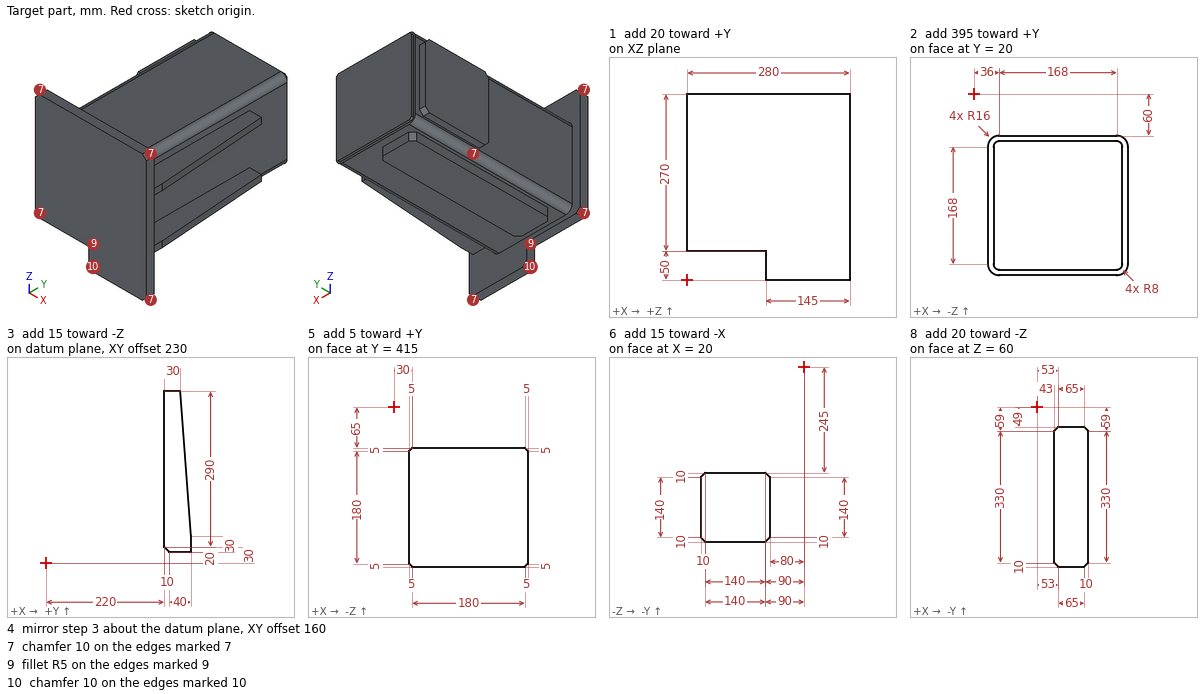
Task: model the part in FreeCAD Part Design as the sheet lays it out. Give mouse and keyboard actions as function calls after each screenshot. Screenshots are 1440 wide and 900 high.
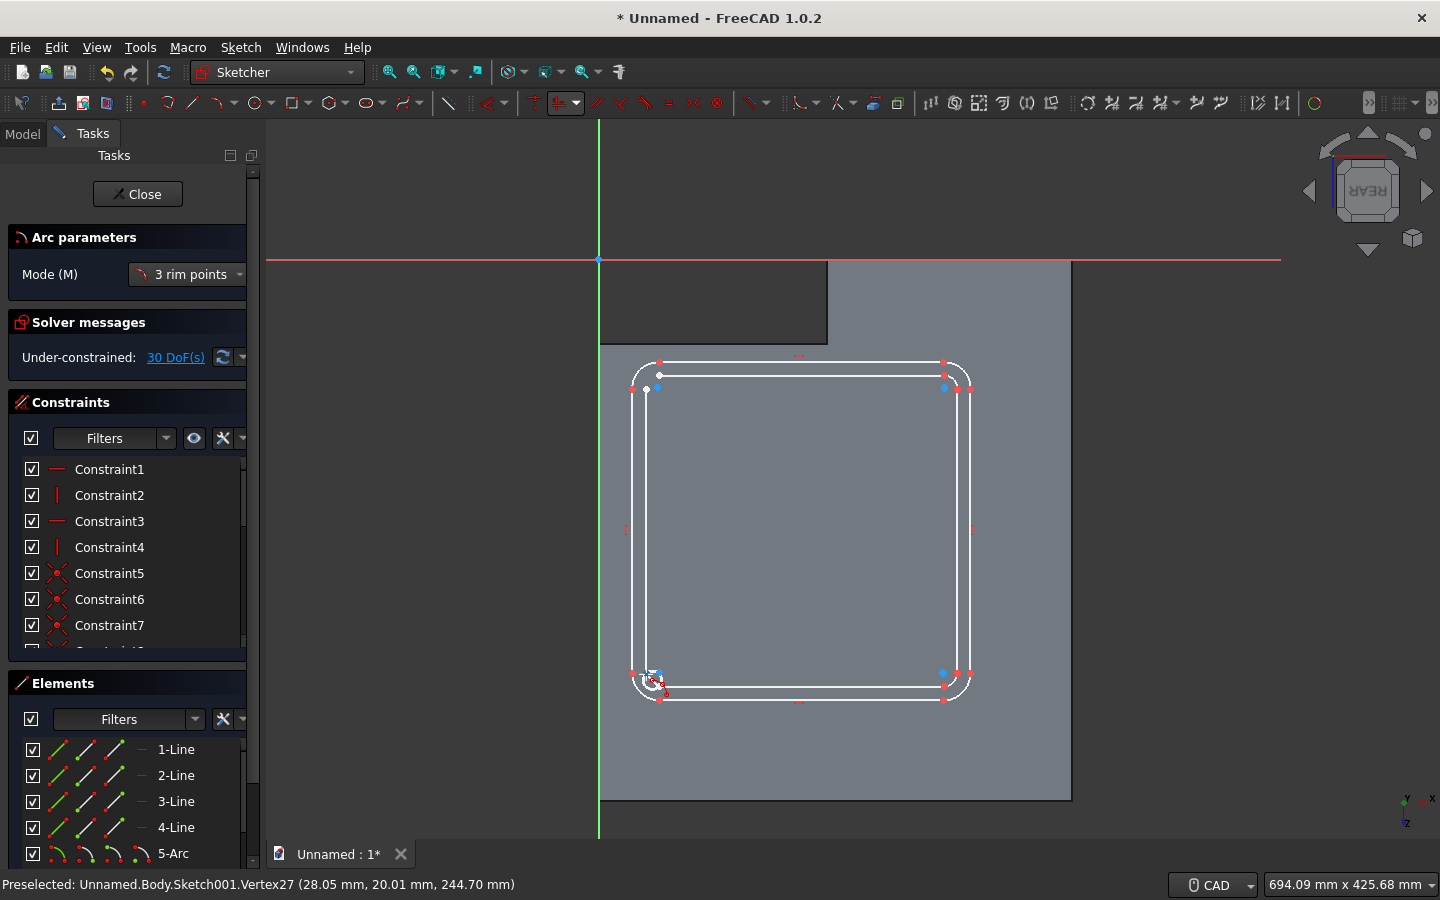
scroll(650, 682, up, 7)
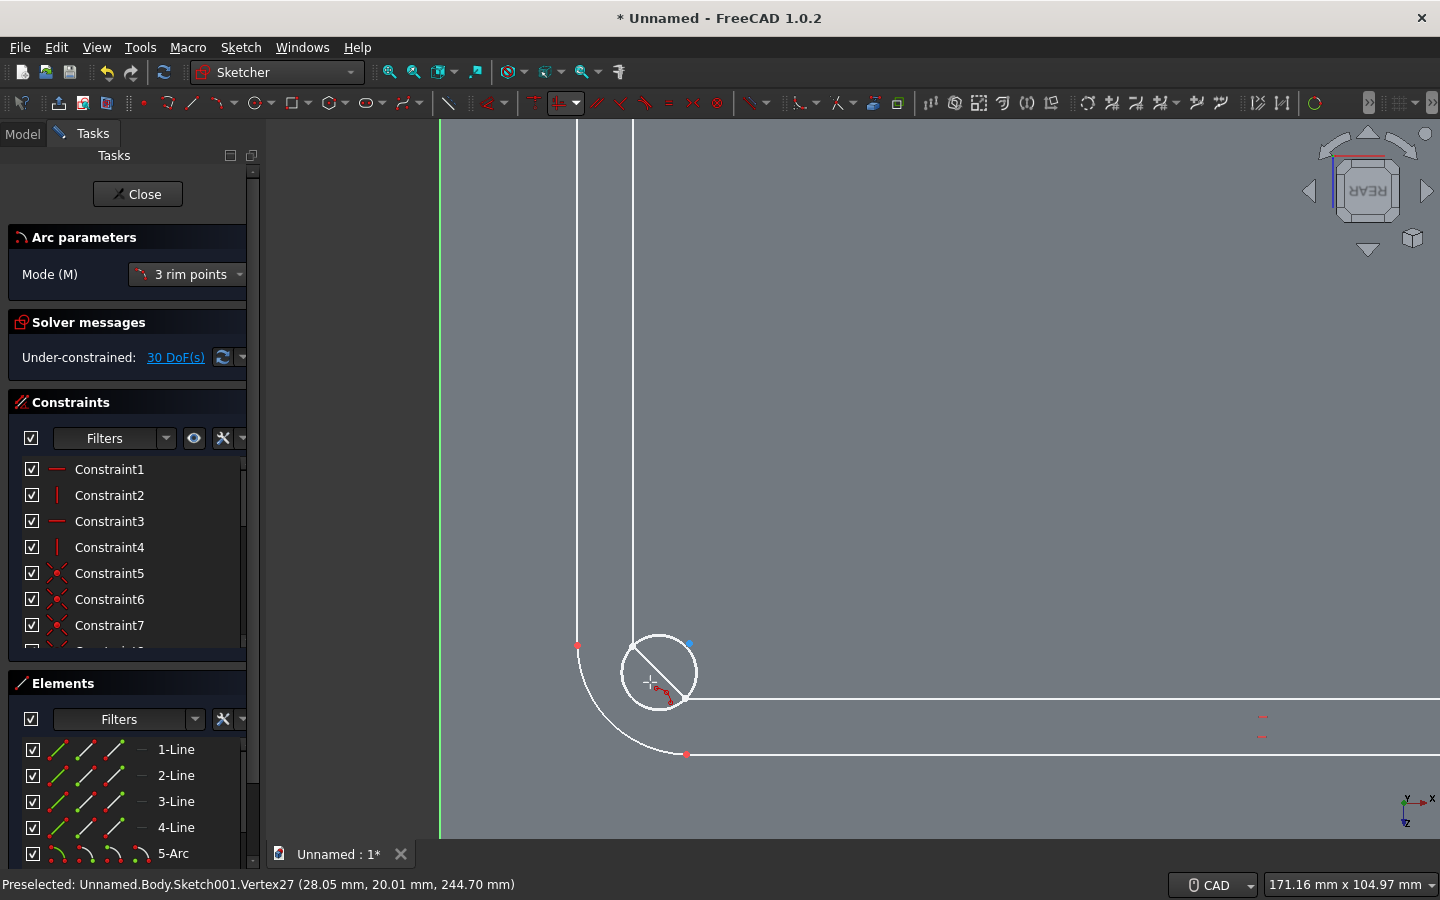
click(649, 680)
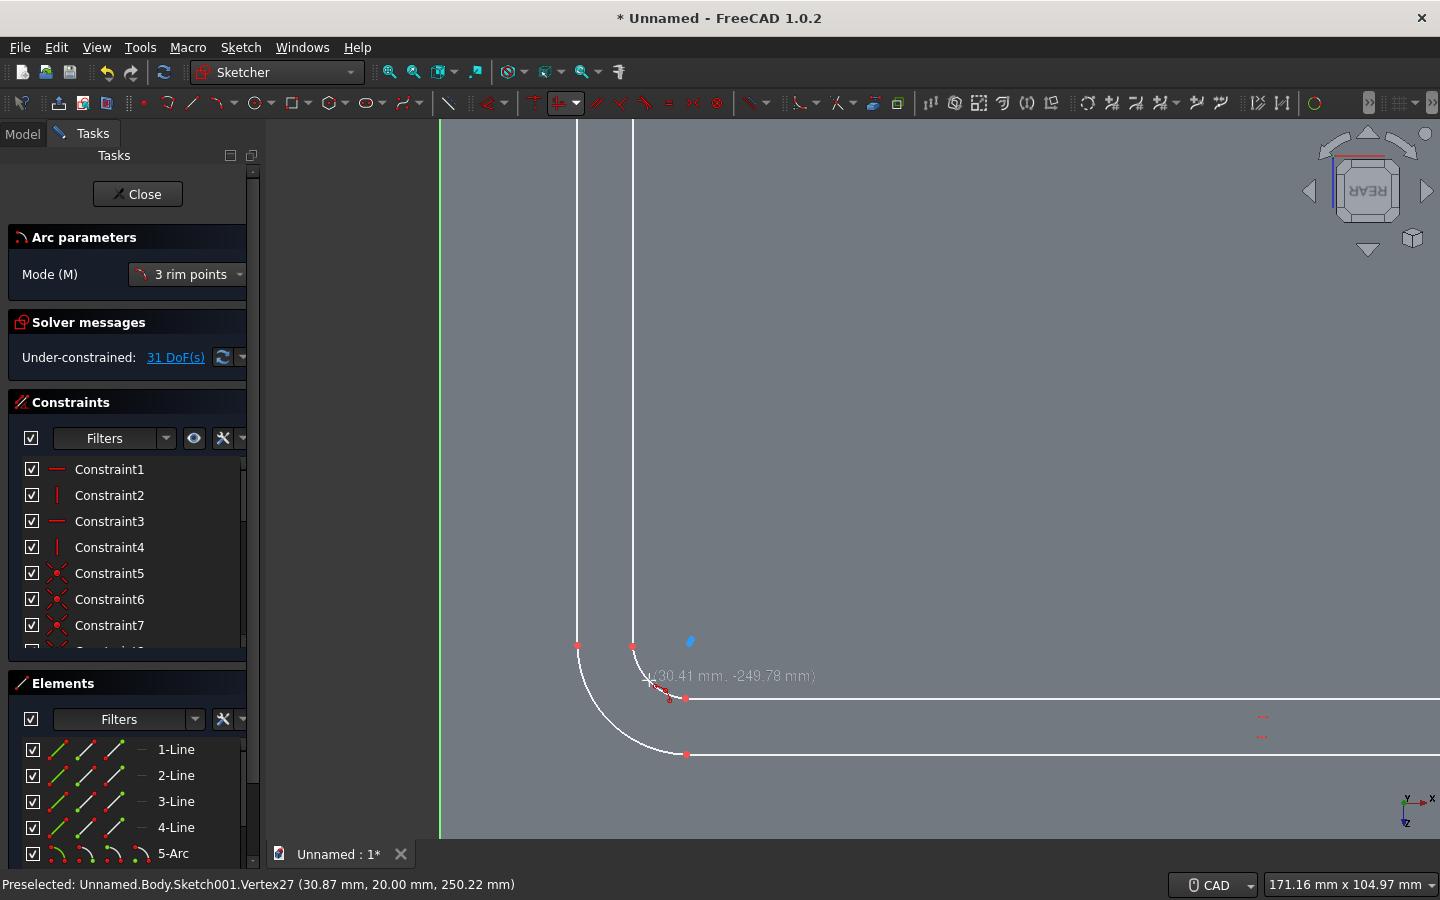
scroll(650, 682, down, 7)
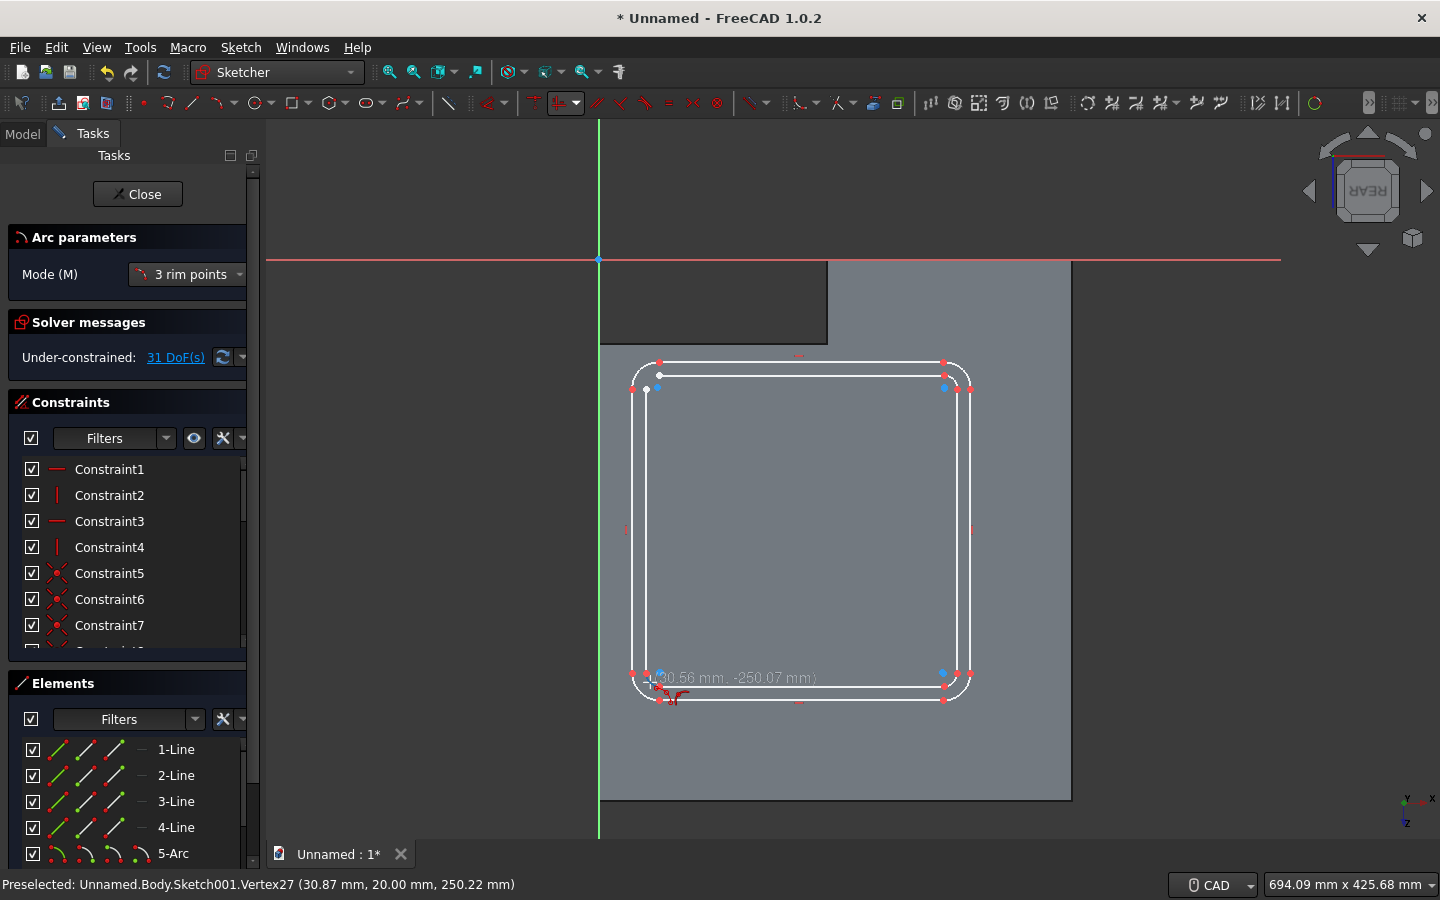
click(646, 390)
click(659, 376)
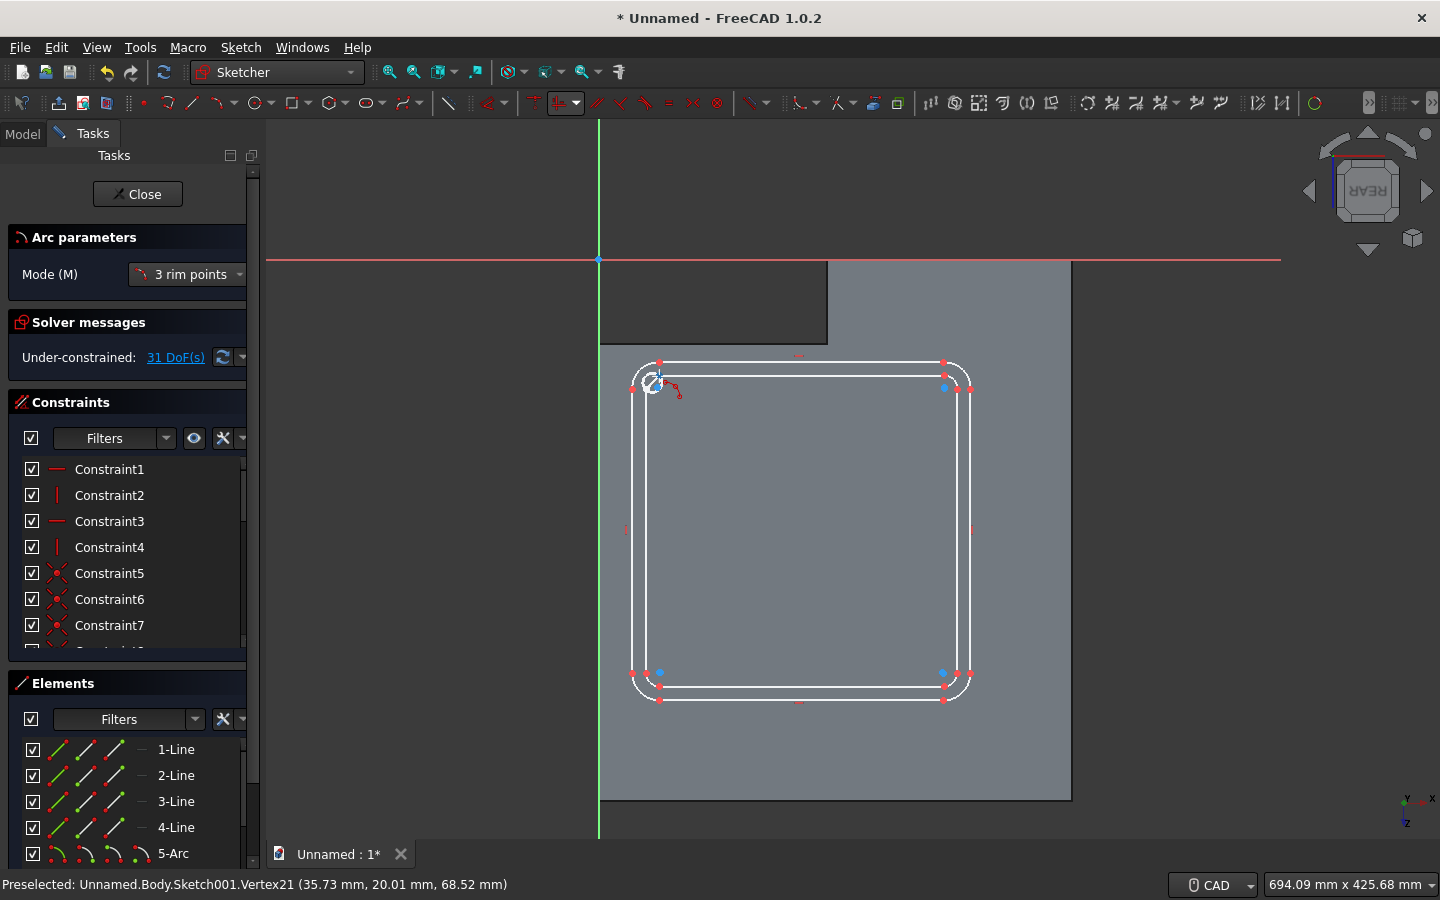
scroll(650, 379, up, 7)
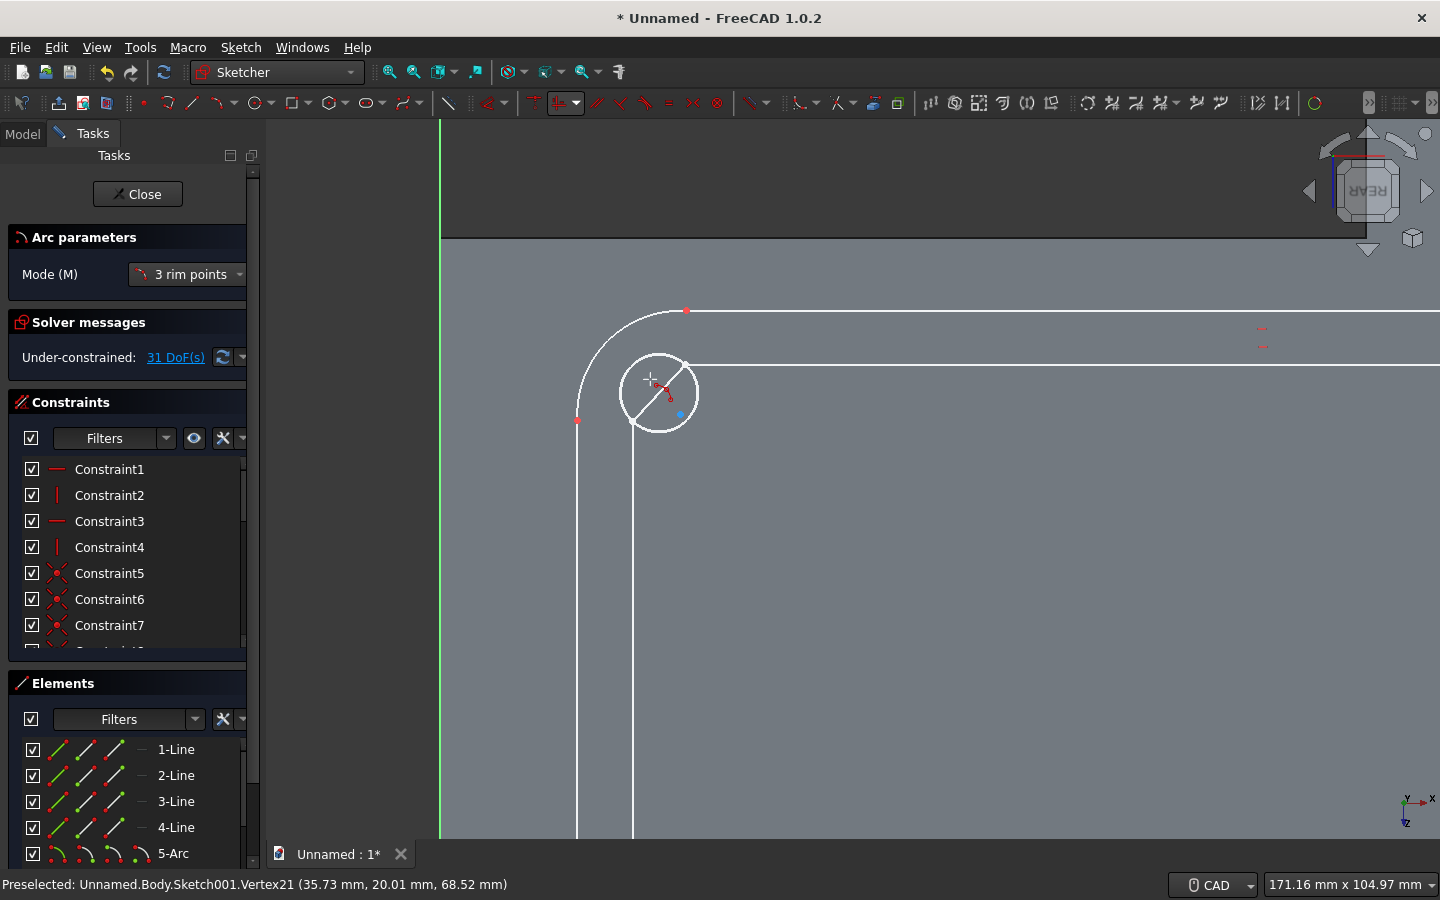
click(649, 377)
key(Escape)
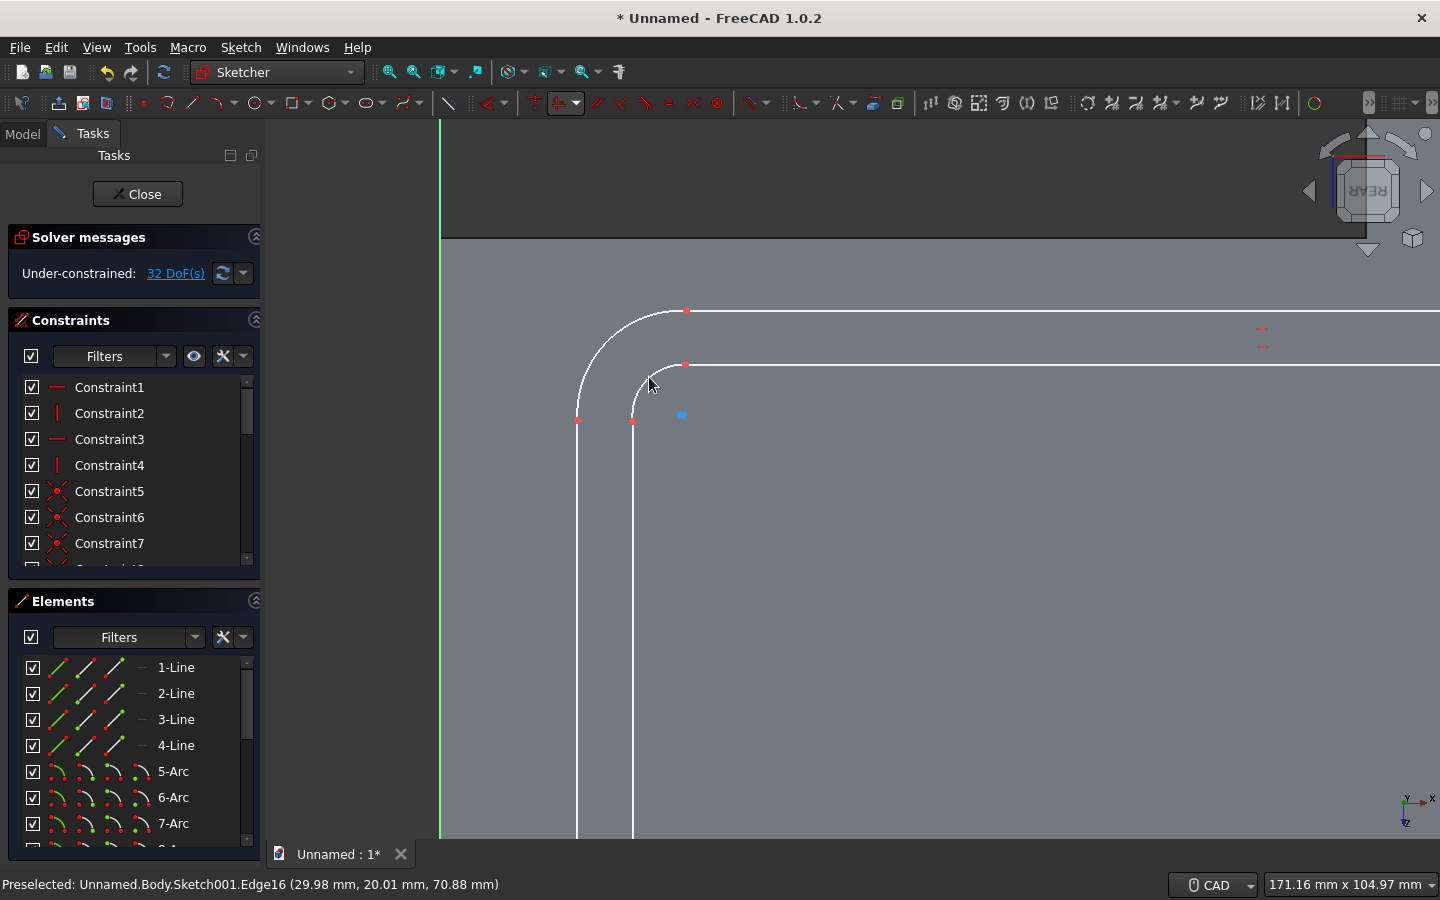
scroll(650, 378, down, 7)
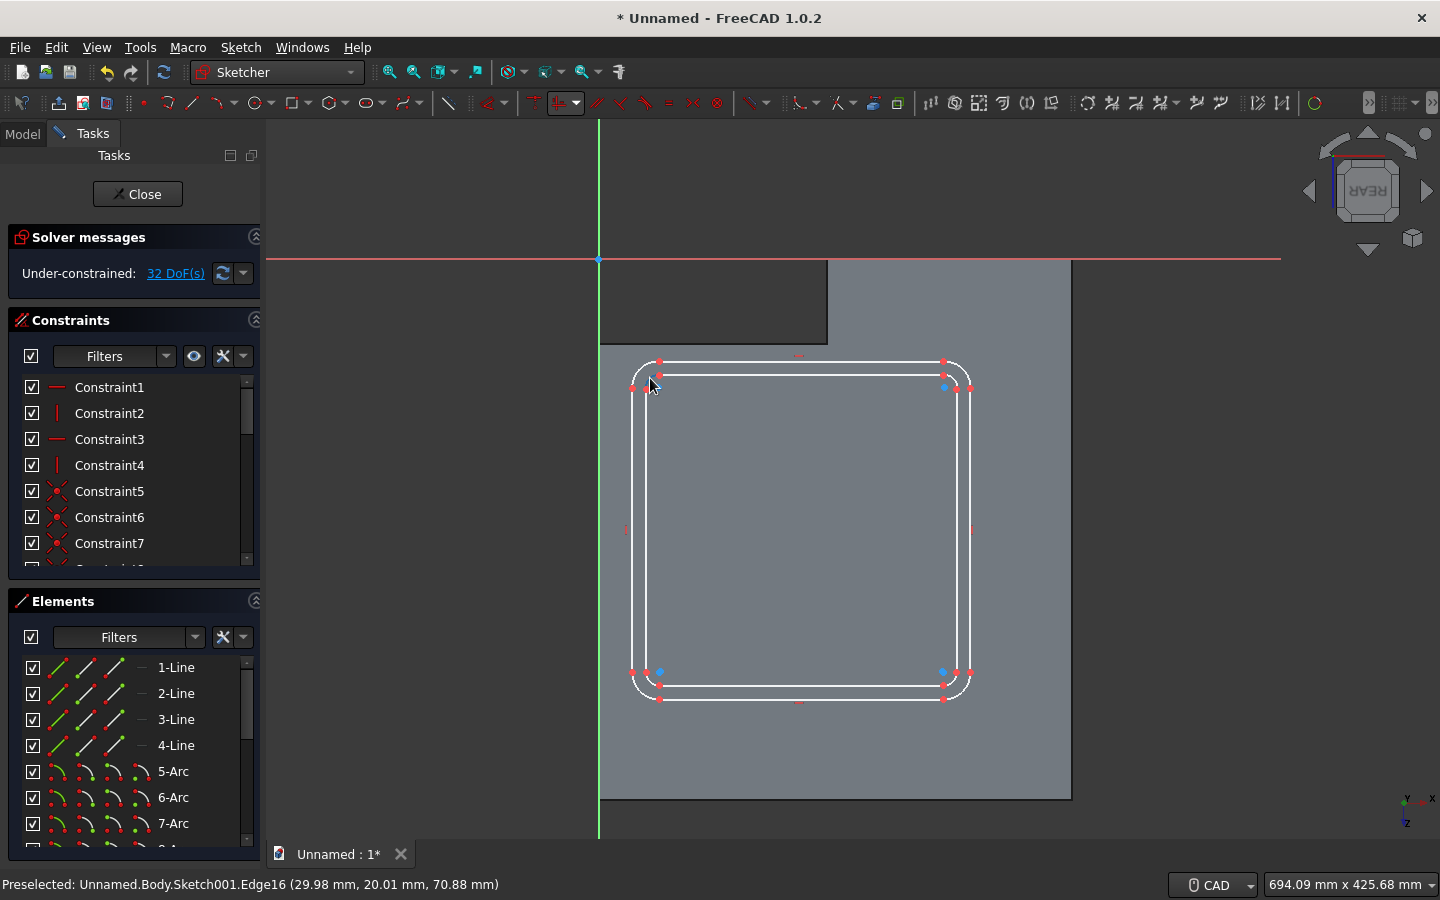
click(745, 362)